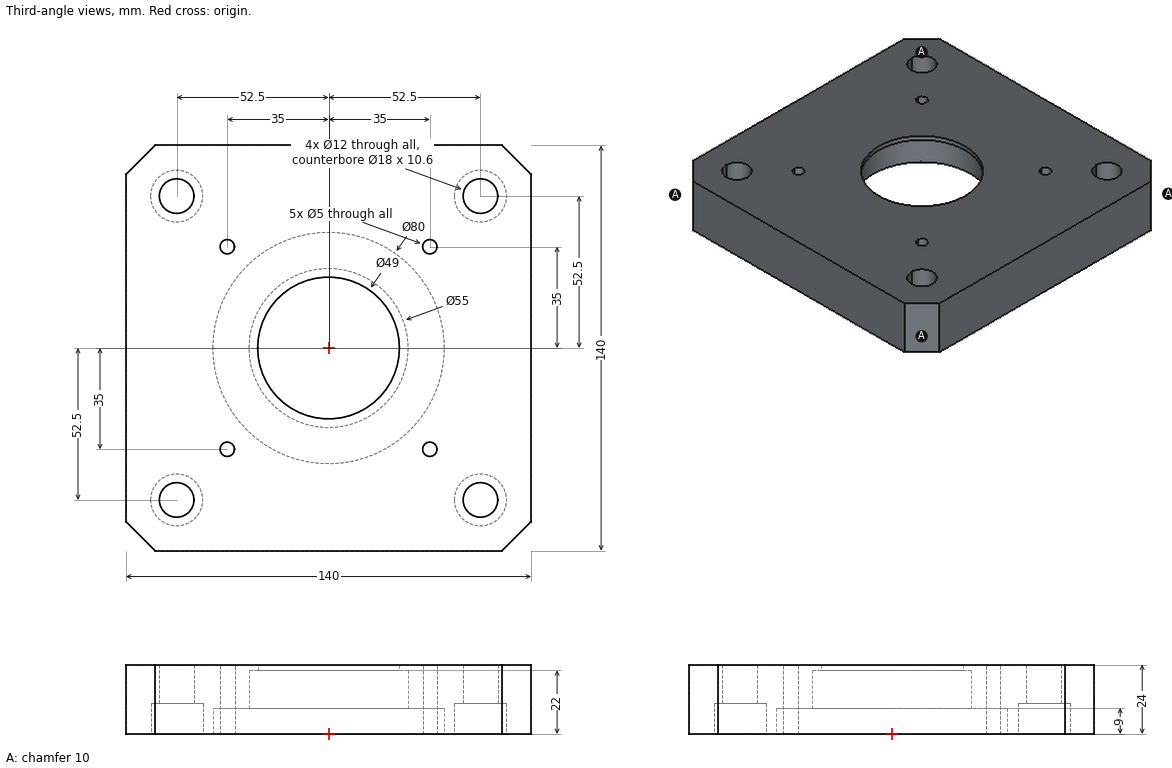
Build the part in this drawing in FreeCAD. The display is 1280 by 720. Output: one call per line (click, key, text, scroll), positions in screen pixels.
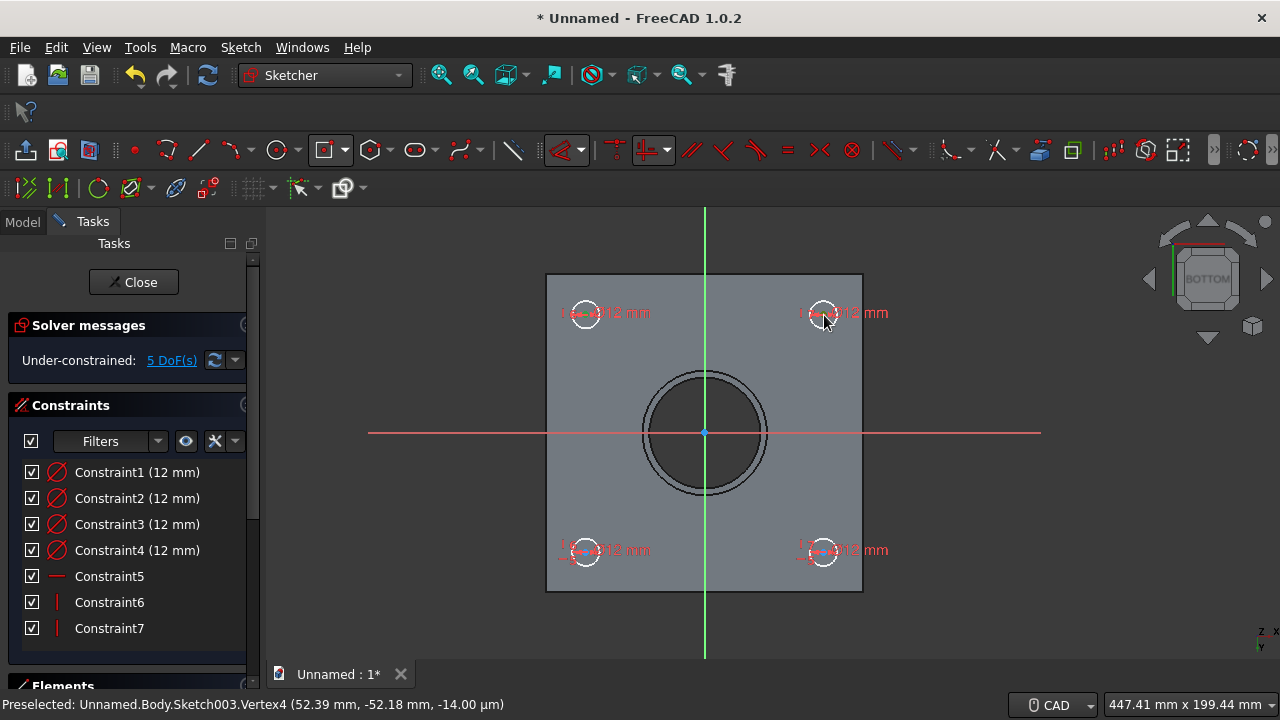
click(670, 150)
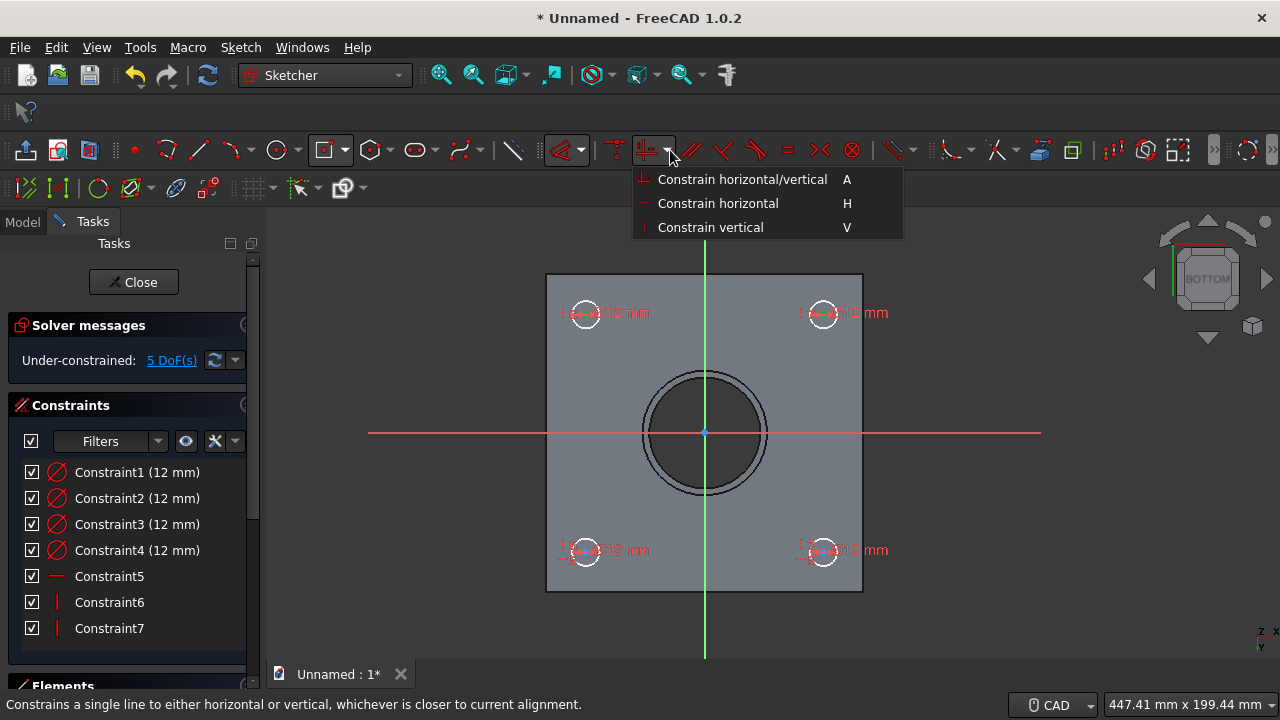
click(768, 203)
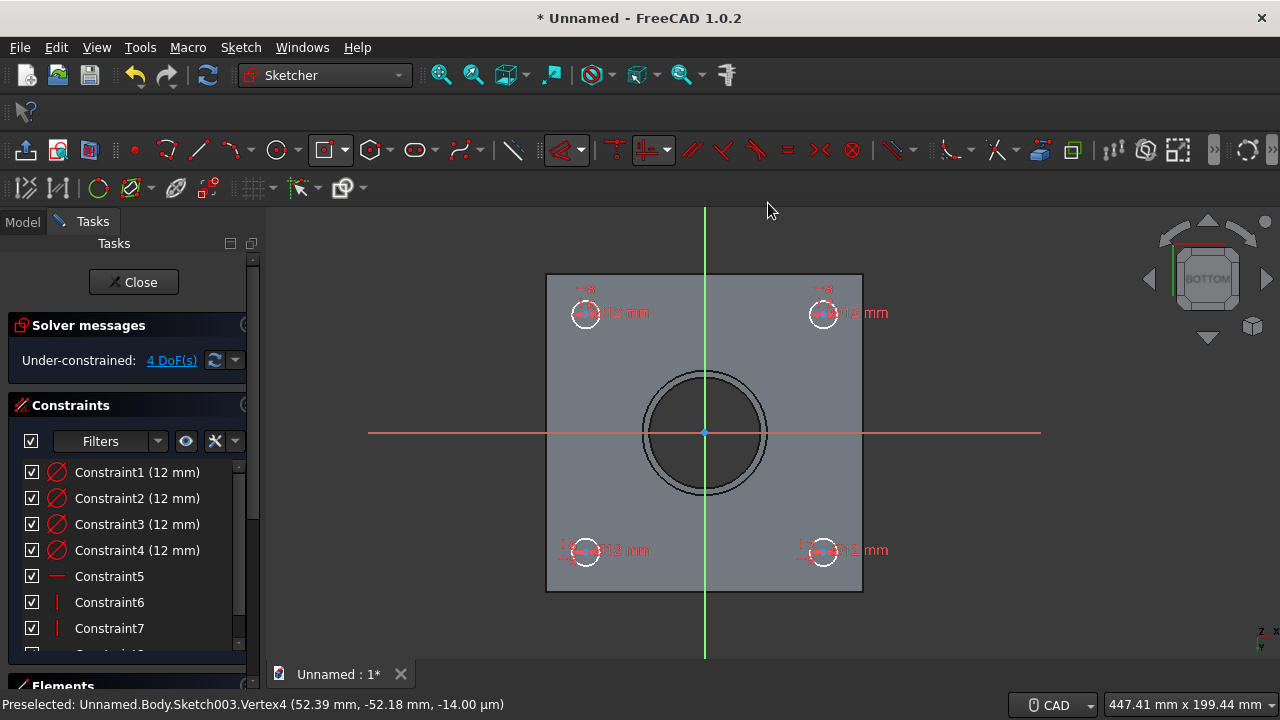
click(560, 150)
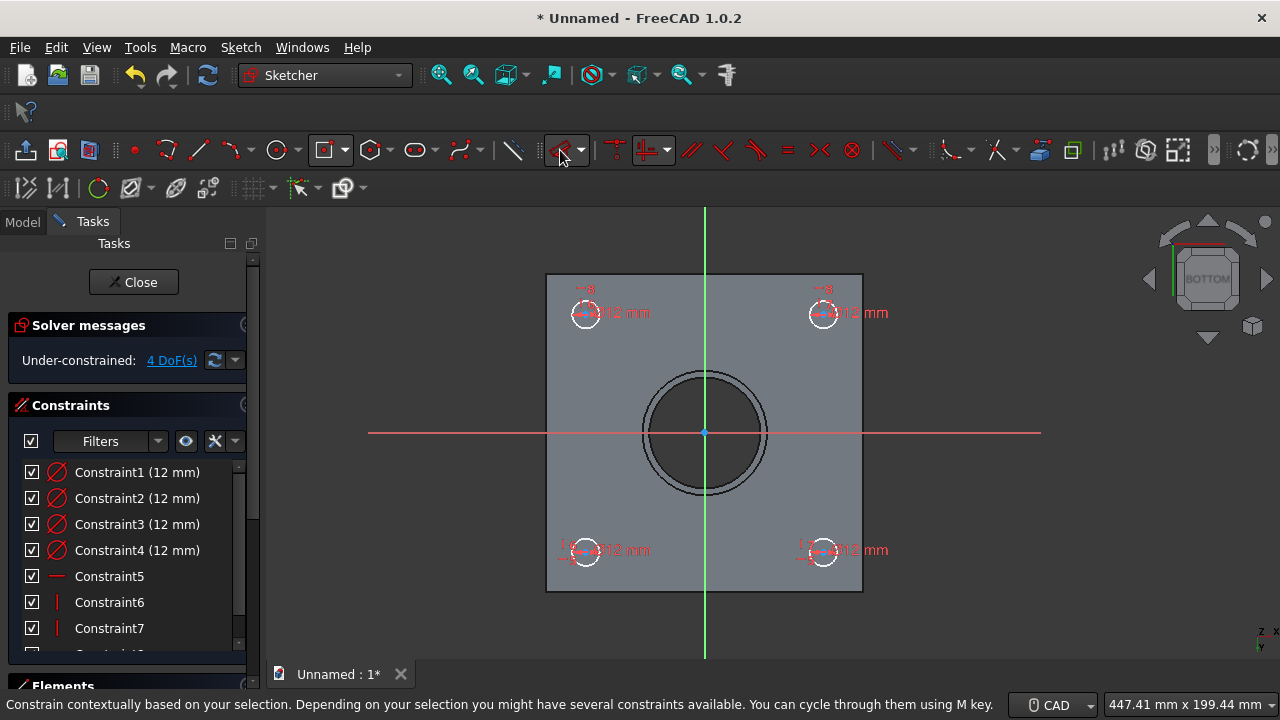
click(824, 552)
click(764, 586)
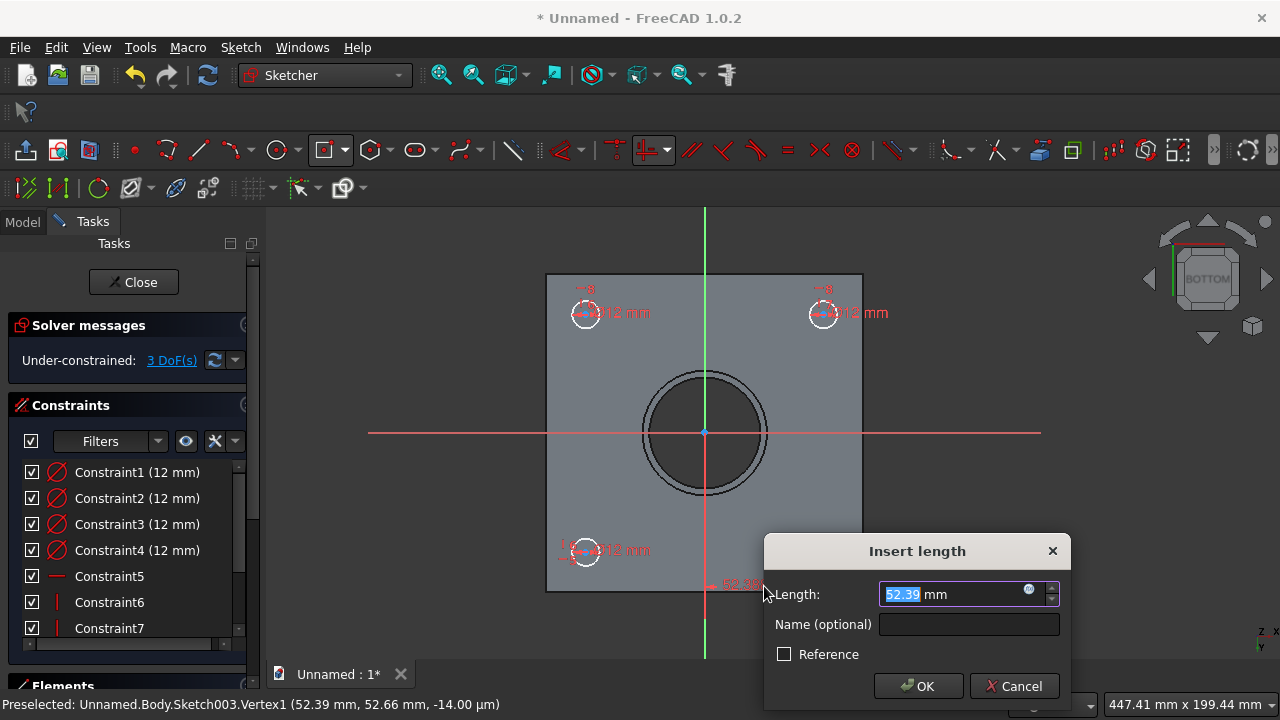
text(52.5)
key(Return)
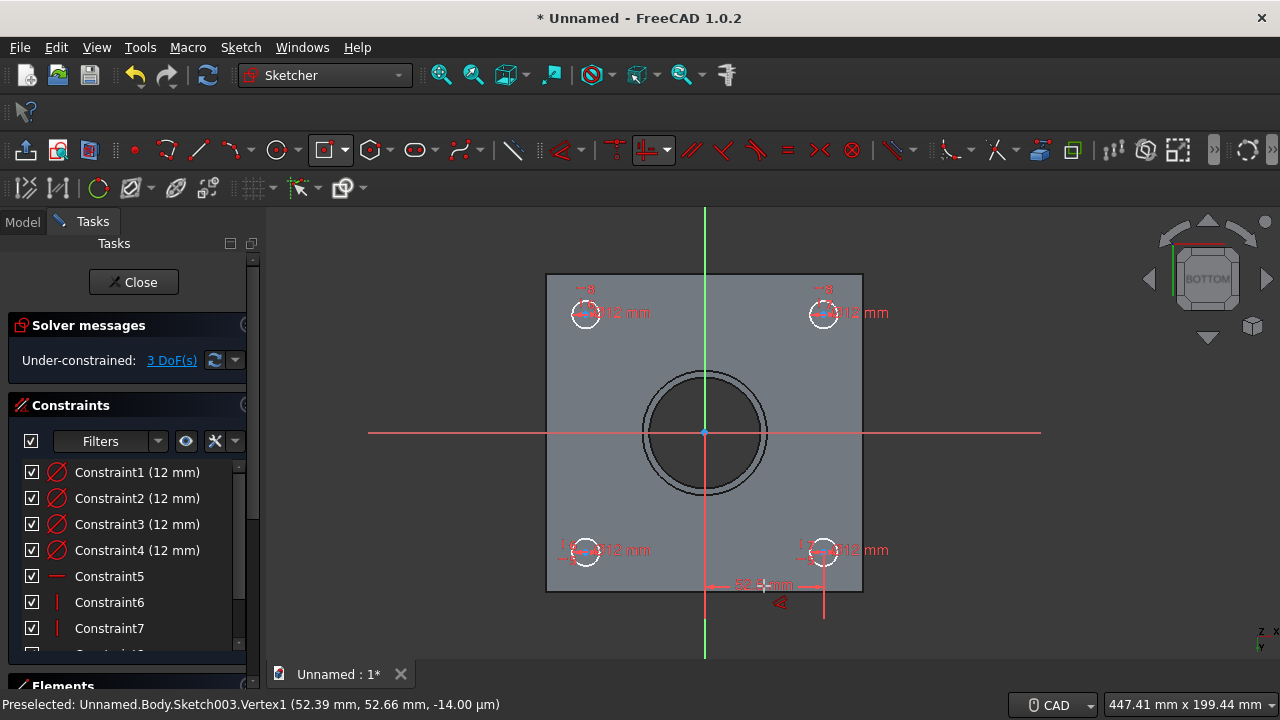
click(824, 552)
click(858, 493)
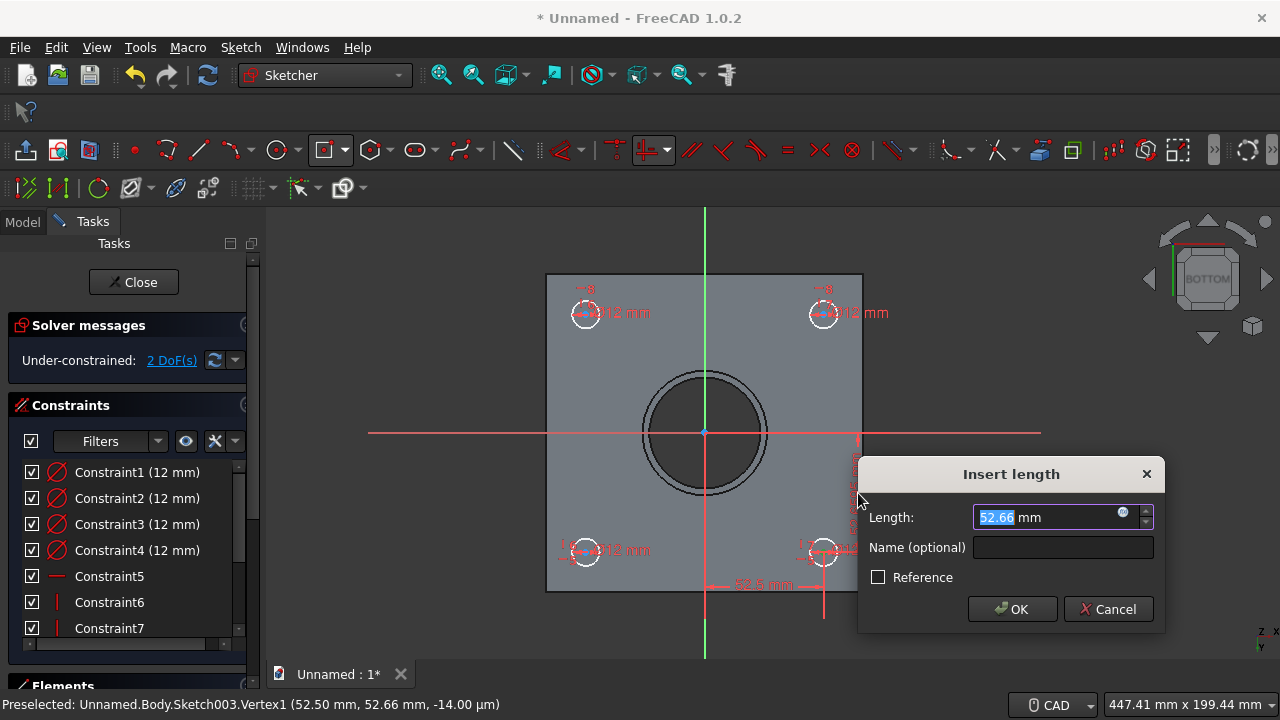
text(52.5)
key(Return)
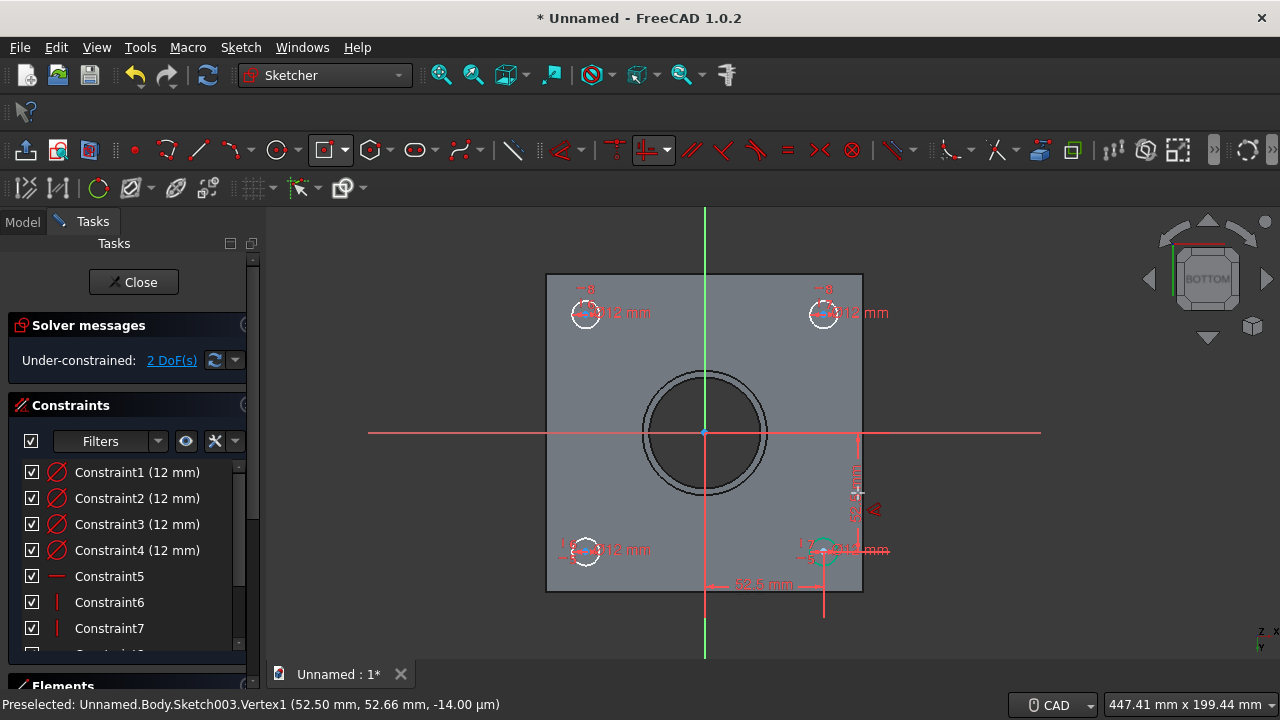
click(586, 552)
click(645, 586)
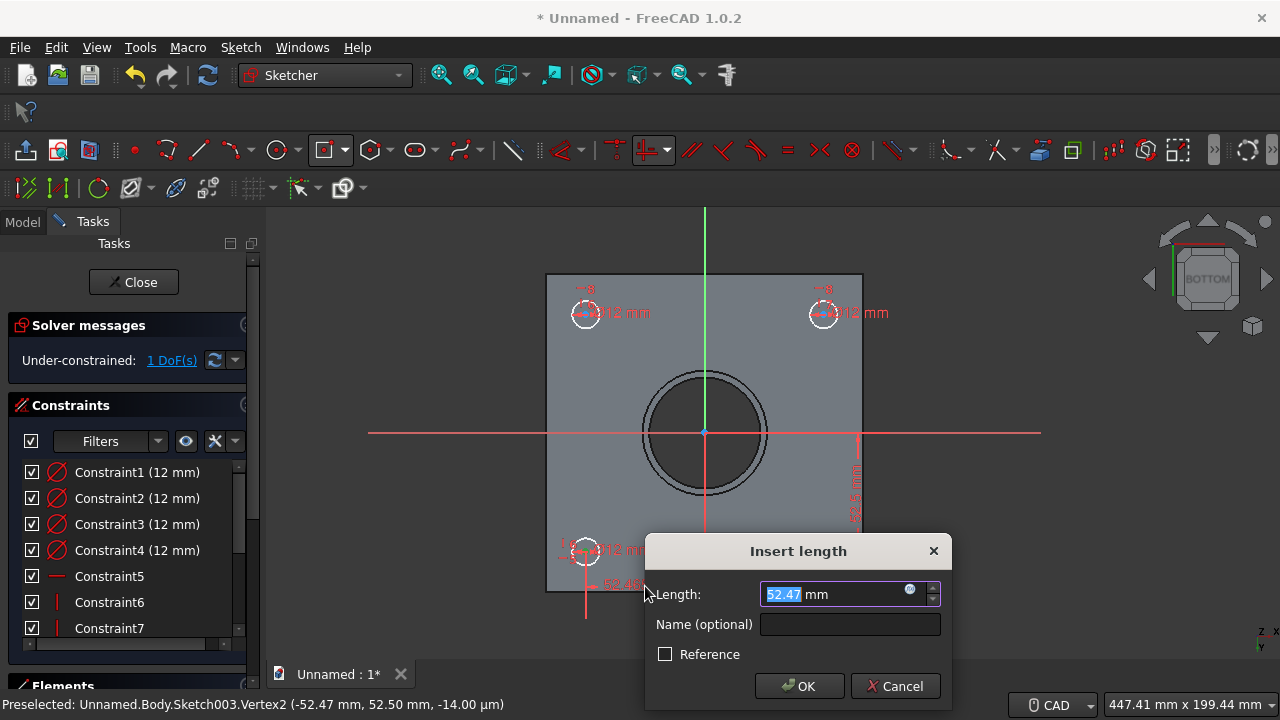
text(52.5)
key(Return)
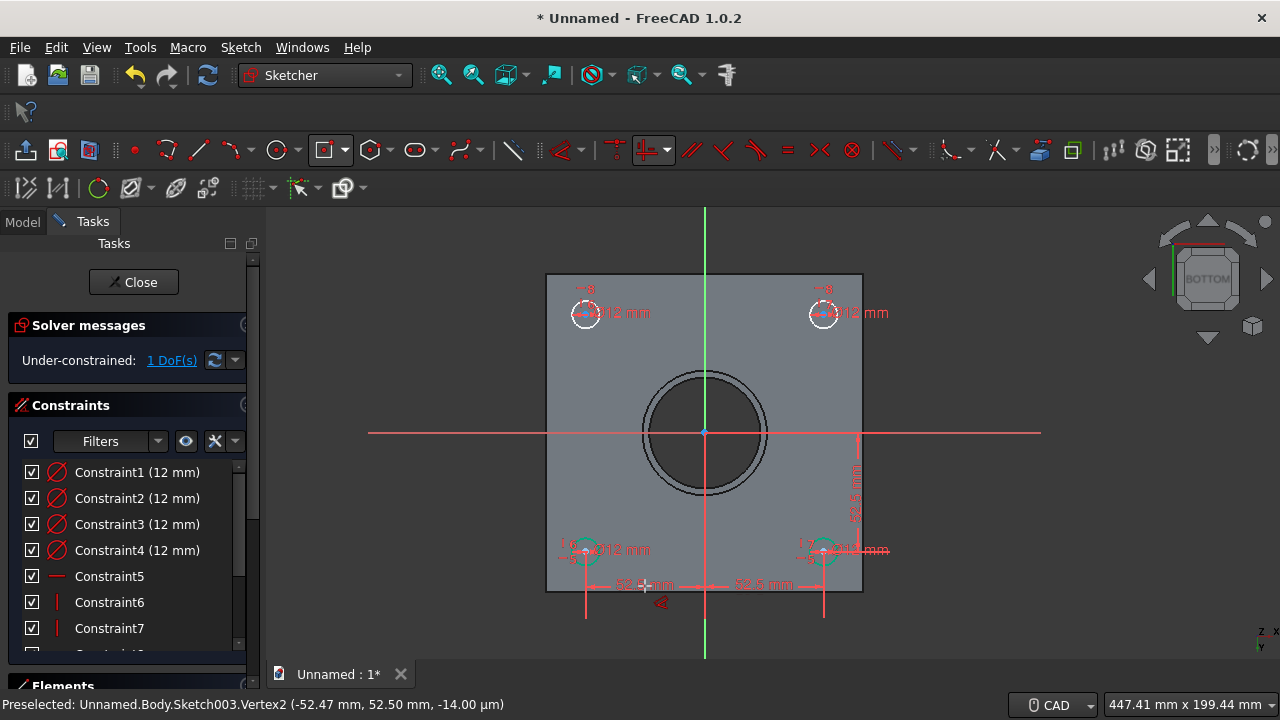
click(586, 315)
click(552, 374)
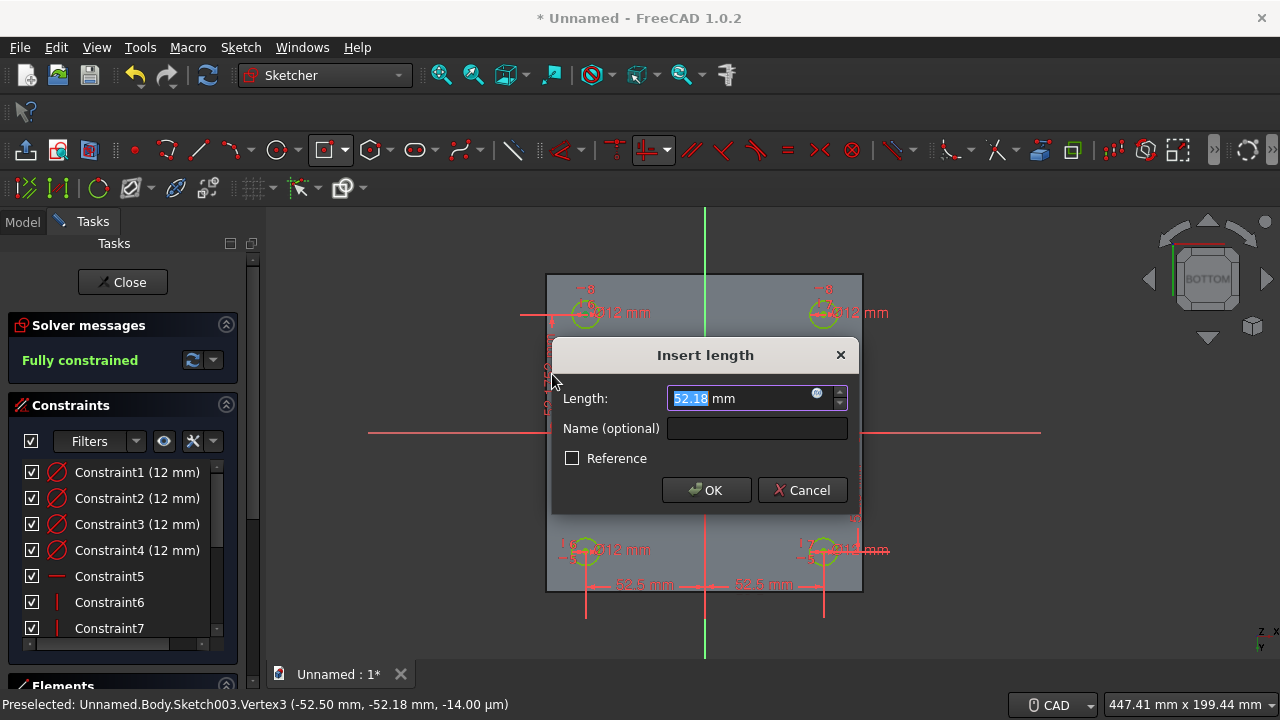
text(52.5)
key(Return)
key(Escape)